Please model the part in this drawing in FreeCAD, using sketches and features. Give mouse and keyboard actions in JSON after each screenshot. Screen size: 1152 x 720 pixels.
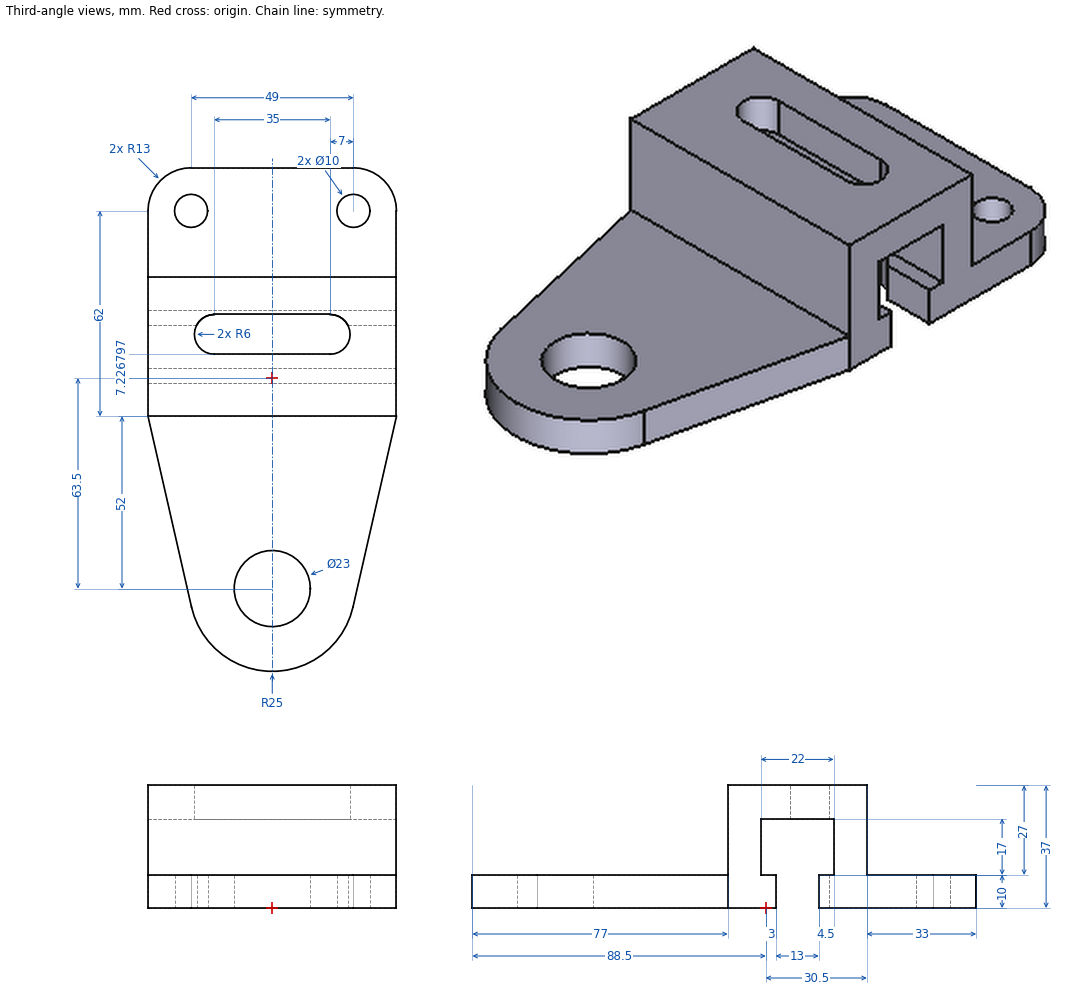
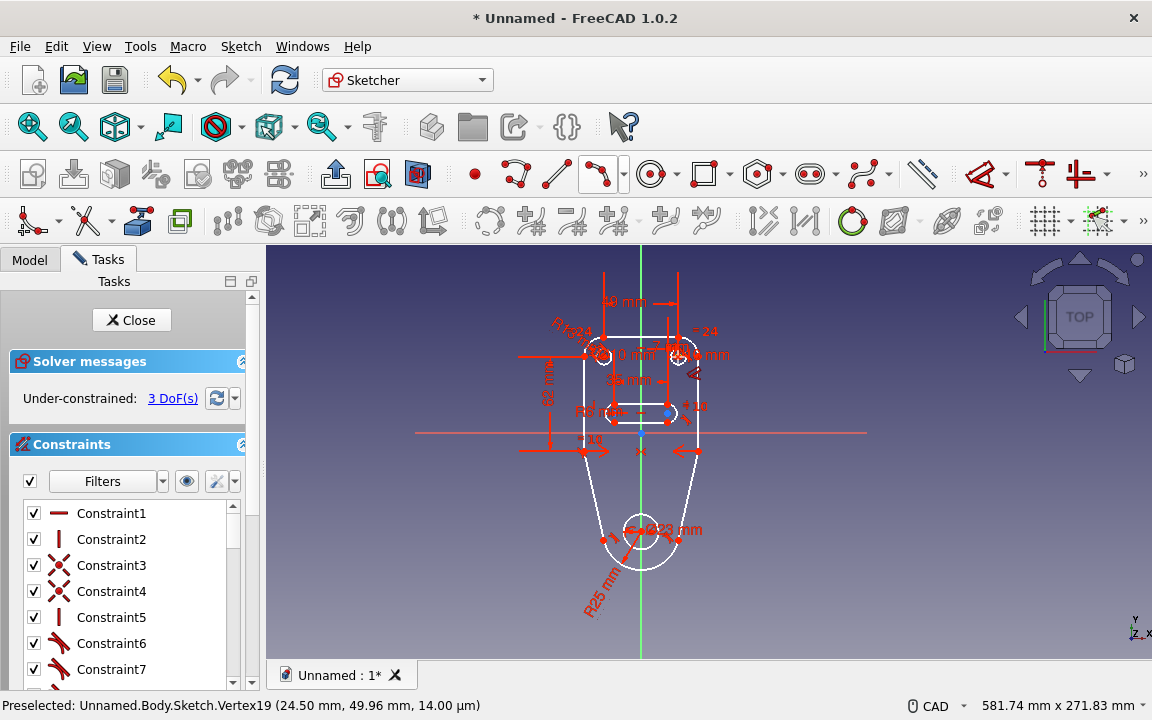
{"action": "left_click", "coordinate": [584, 451]}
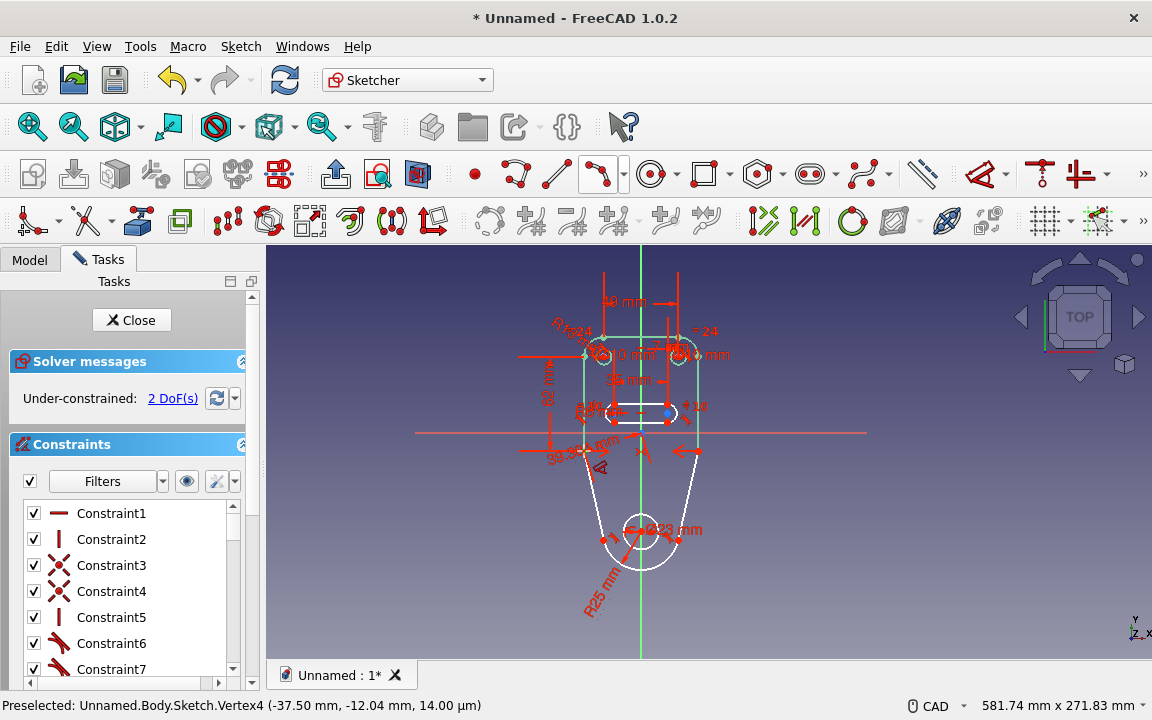
{"action": "left_click", "coordinate": [641, 532]}
{"action": "left_click", "coordinate": [550, 492]}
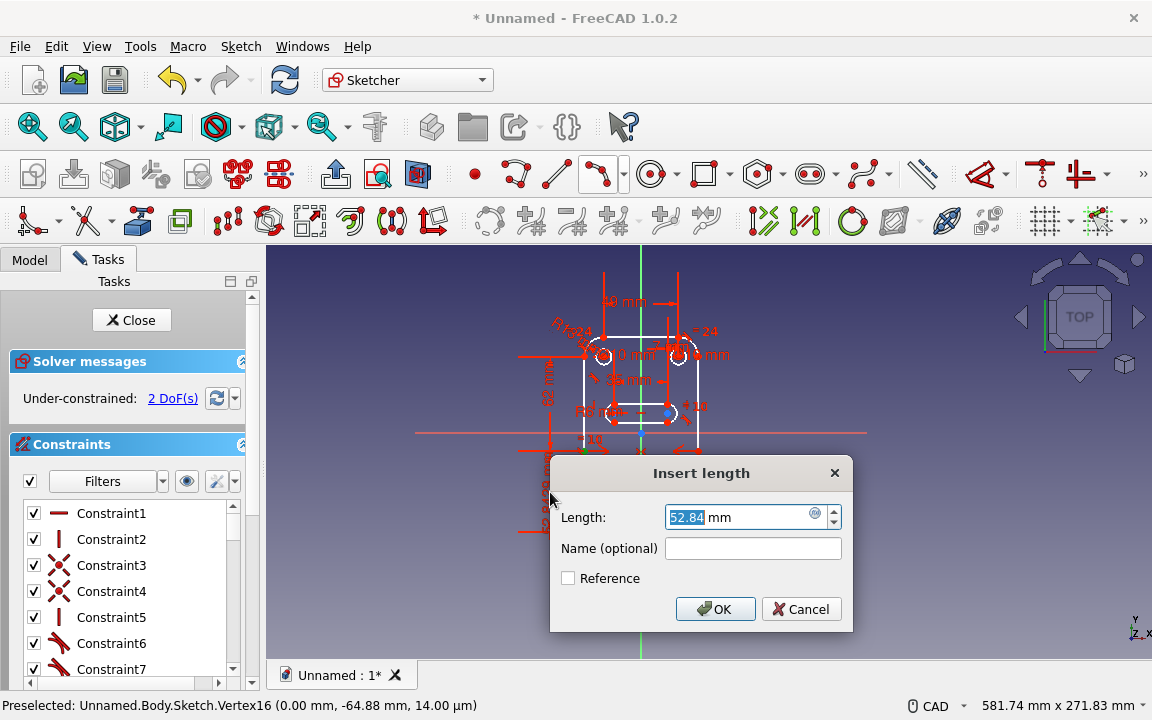
{"action": "type", "text": "52"}
{"action": "key", "text": "Return"}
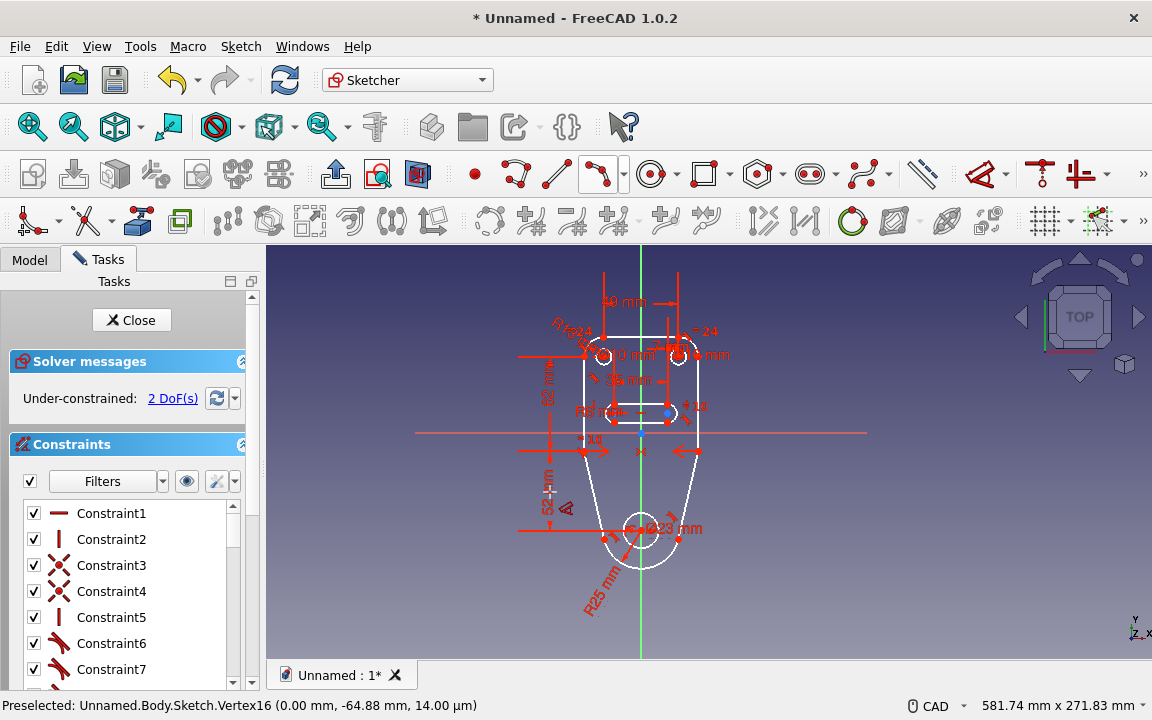
{"action": "left_click", "coordinate": [641, 531]}
{"action": "left_click", "coordinate": [675, 482]}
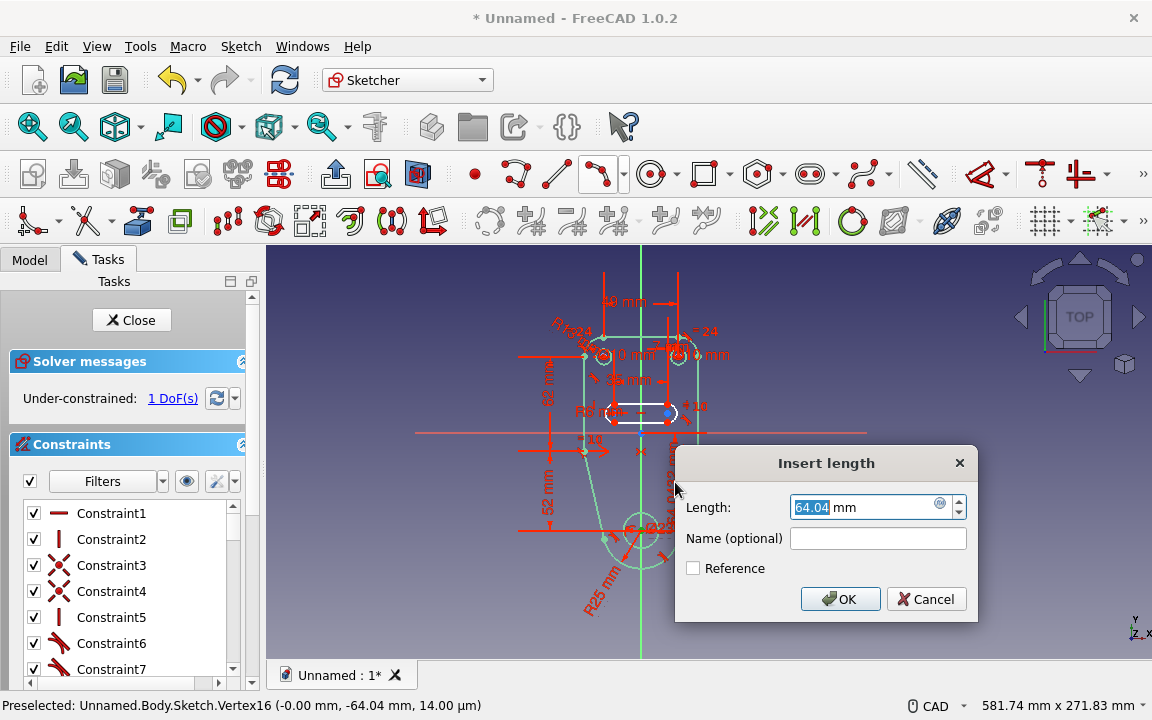
{"action": "type", "text": "63.5"}
{"action": "key", "text": "Return"}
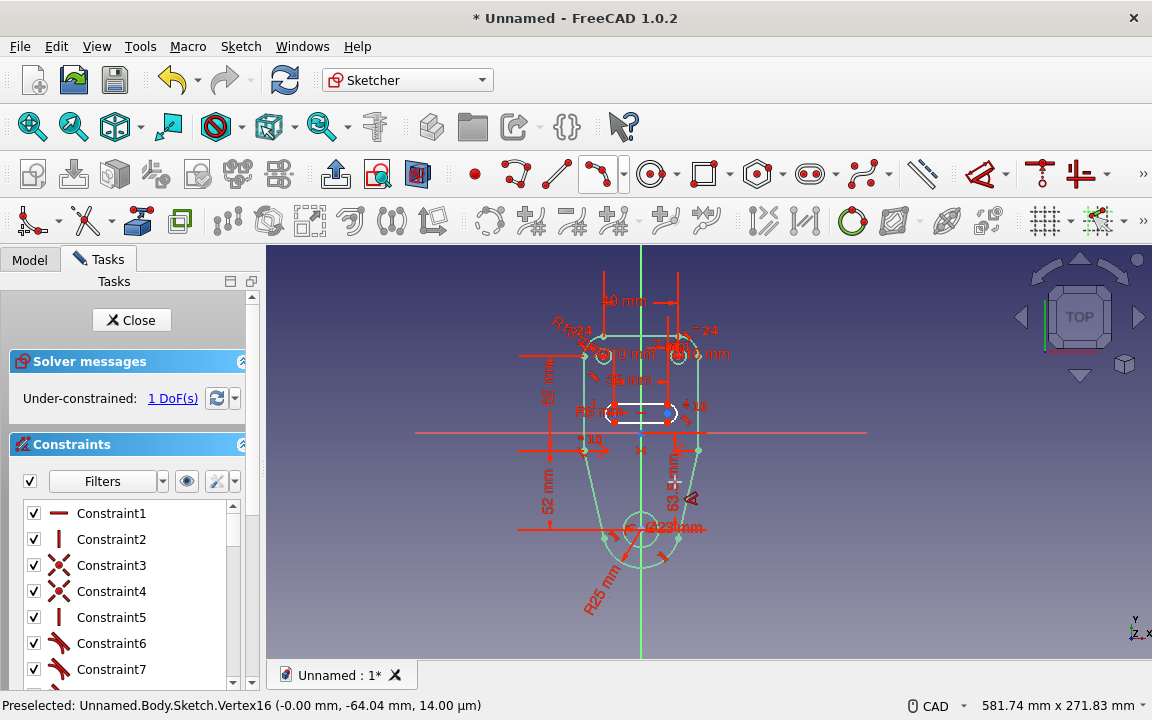
{"action": "scroll", "coordinate": [614, 423], "scroll_direction": "up", "scroll_amount": 7}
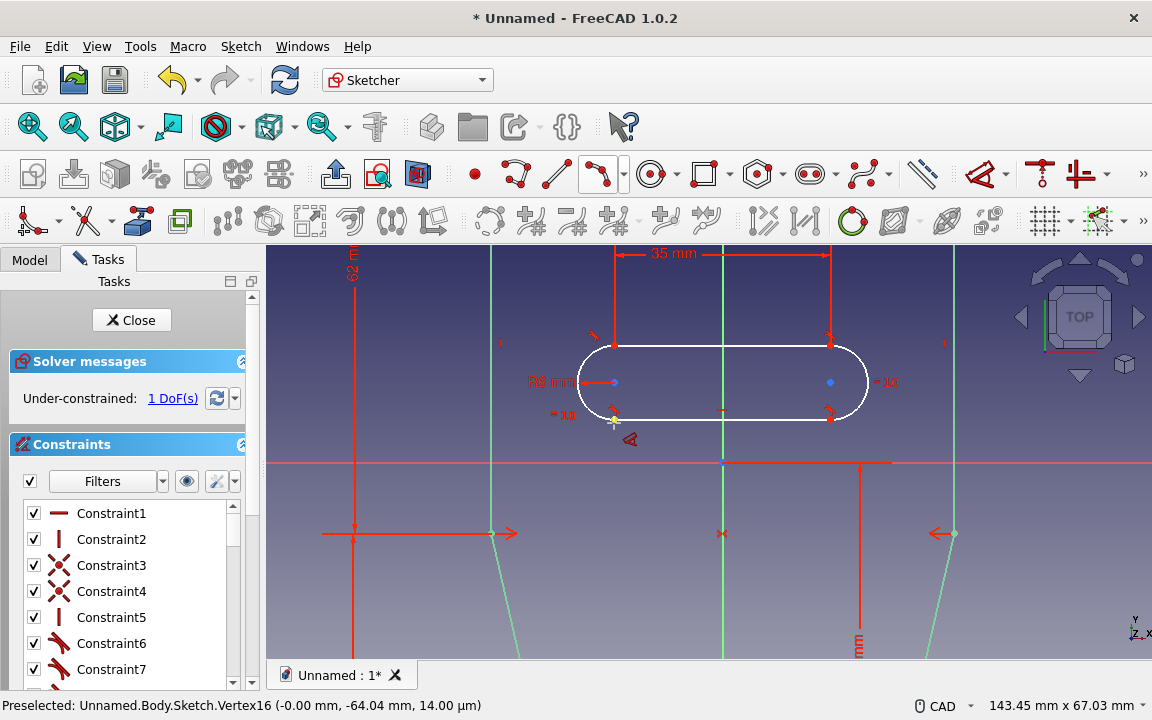
{"action": "left_click", "coordinate": [615, 420]}
{"action": "left_click", "coordinate": [581, 441]}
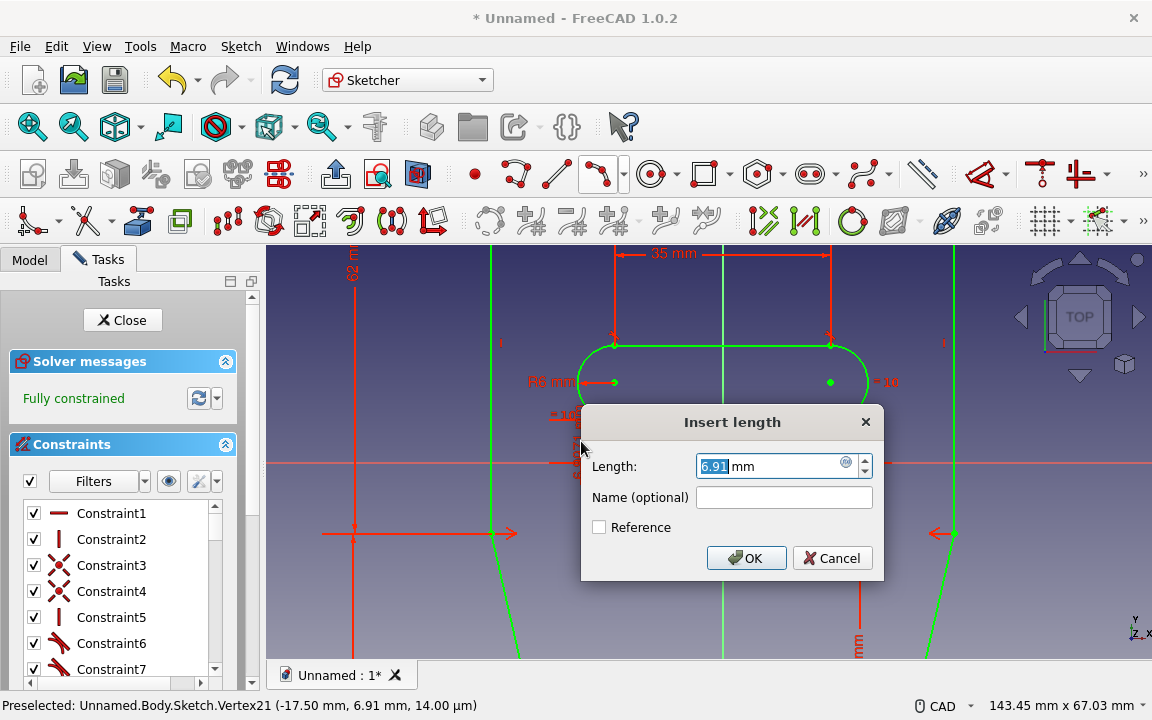
{"action": "type", "text": "7.226797"}
{"action": "key", "text": "Return"}
{"action": "key", "text": "Escape"}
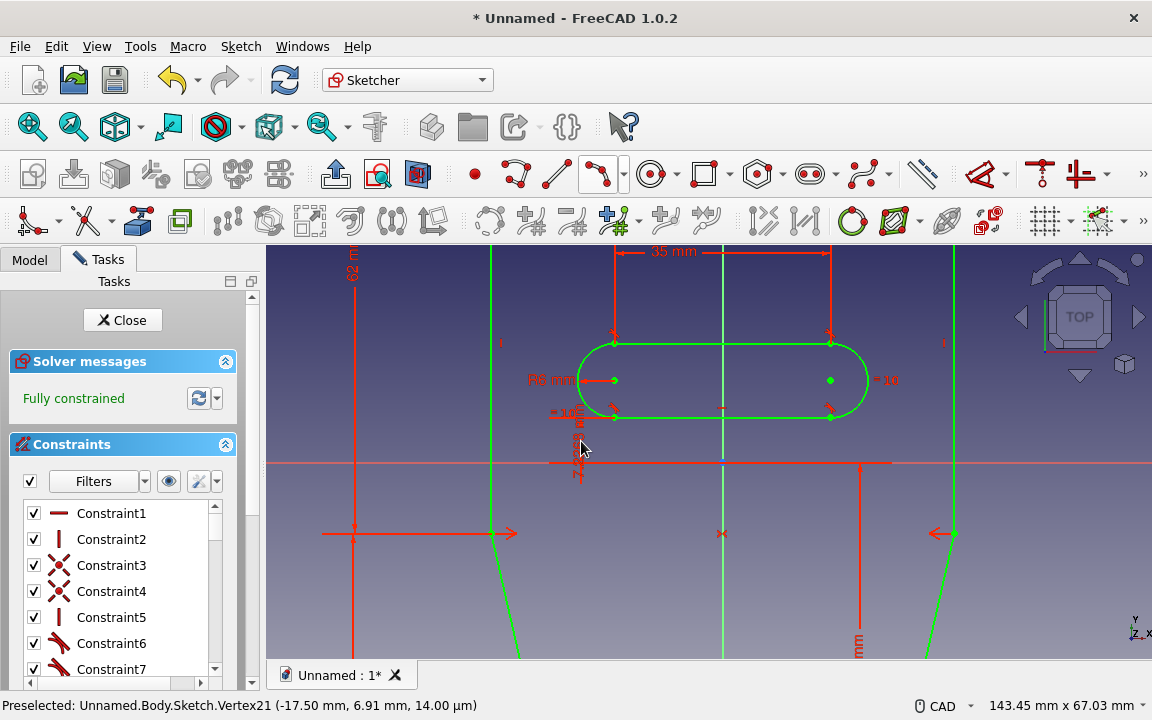
{"action": "left_click", "coordinate": [123, 320]}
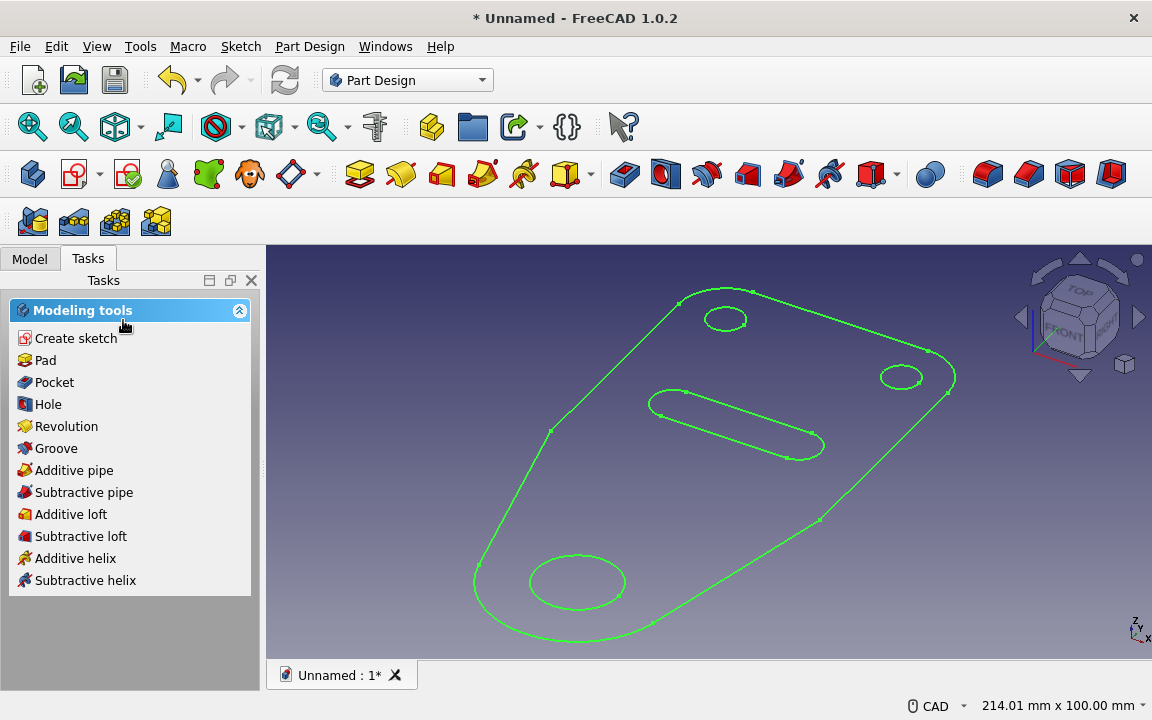
{"action": "left_click", "coordinate": [360, 174]}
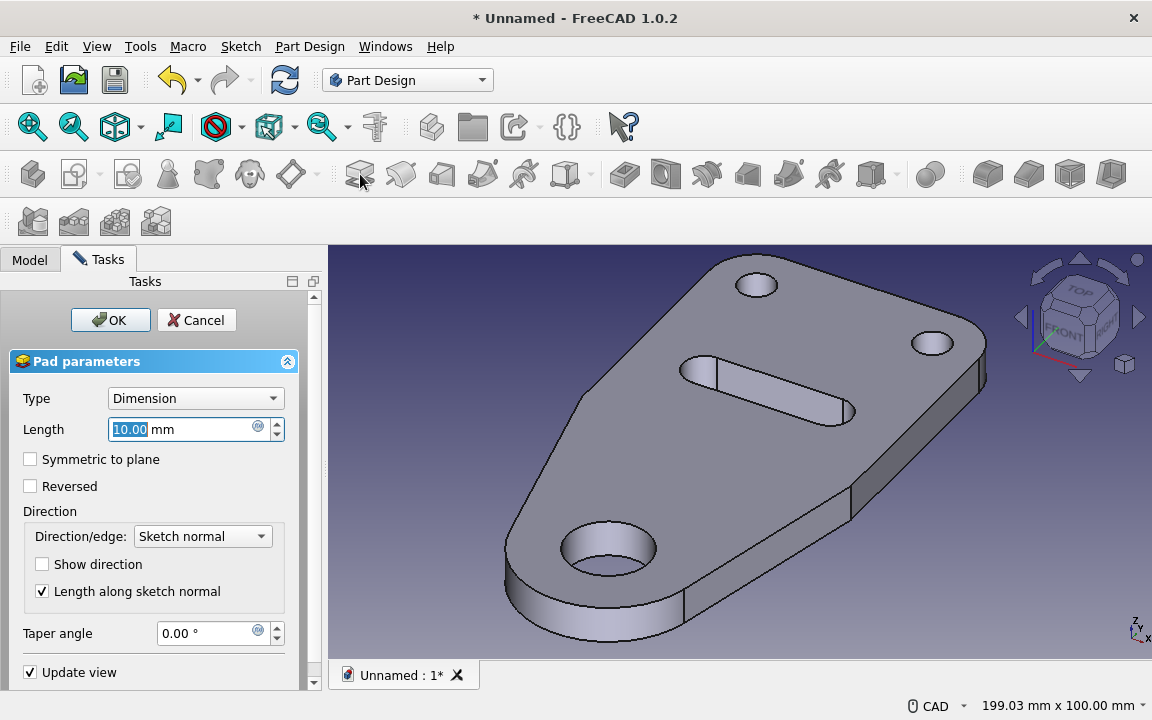
{"action": "type", "text": "37"}
{"action": "key", "text": "Tab"}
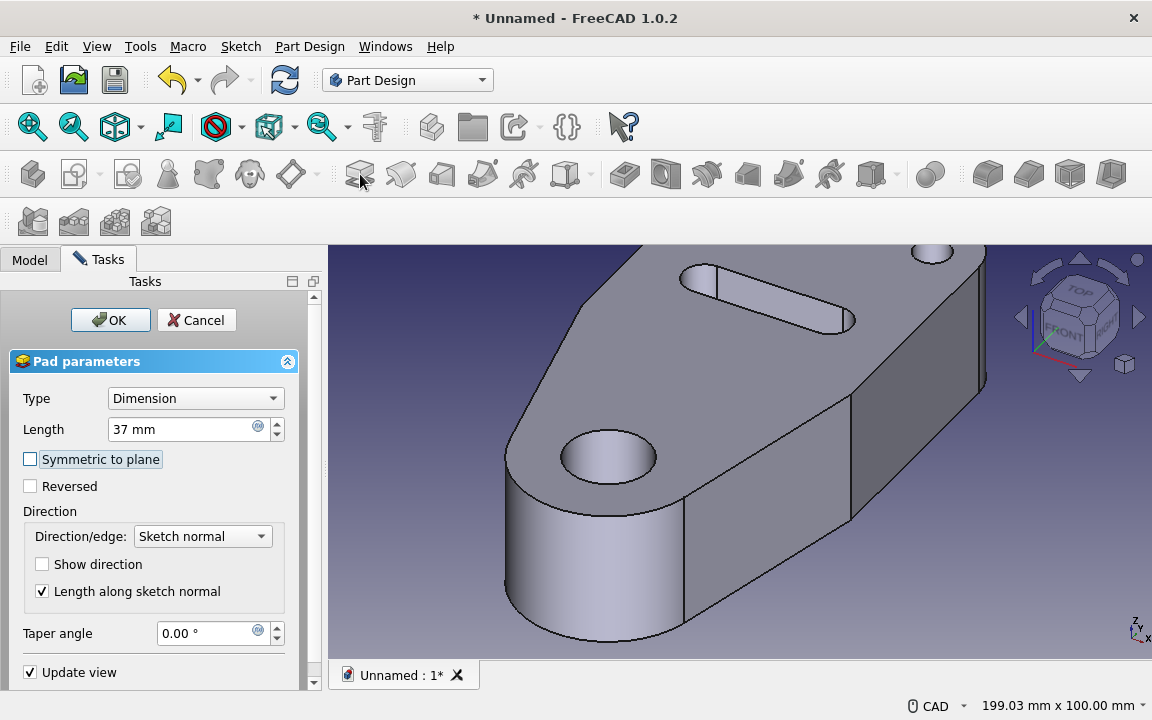
{"action": "left_click", "coordinate": [111, 320]}